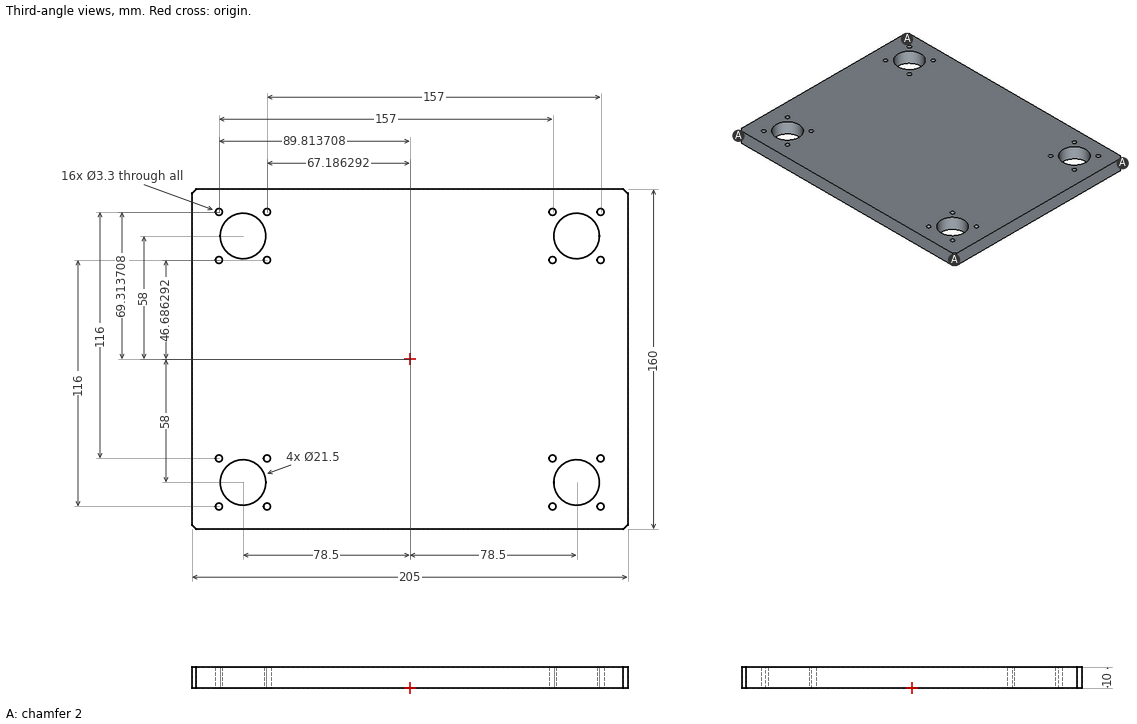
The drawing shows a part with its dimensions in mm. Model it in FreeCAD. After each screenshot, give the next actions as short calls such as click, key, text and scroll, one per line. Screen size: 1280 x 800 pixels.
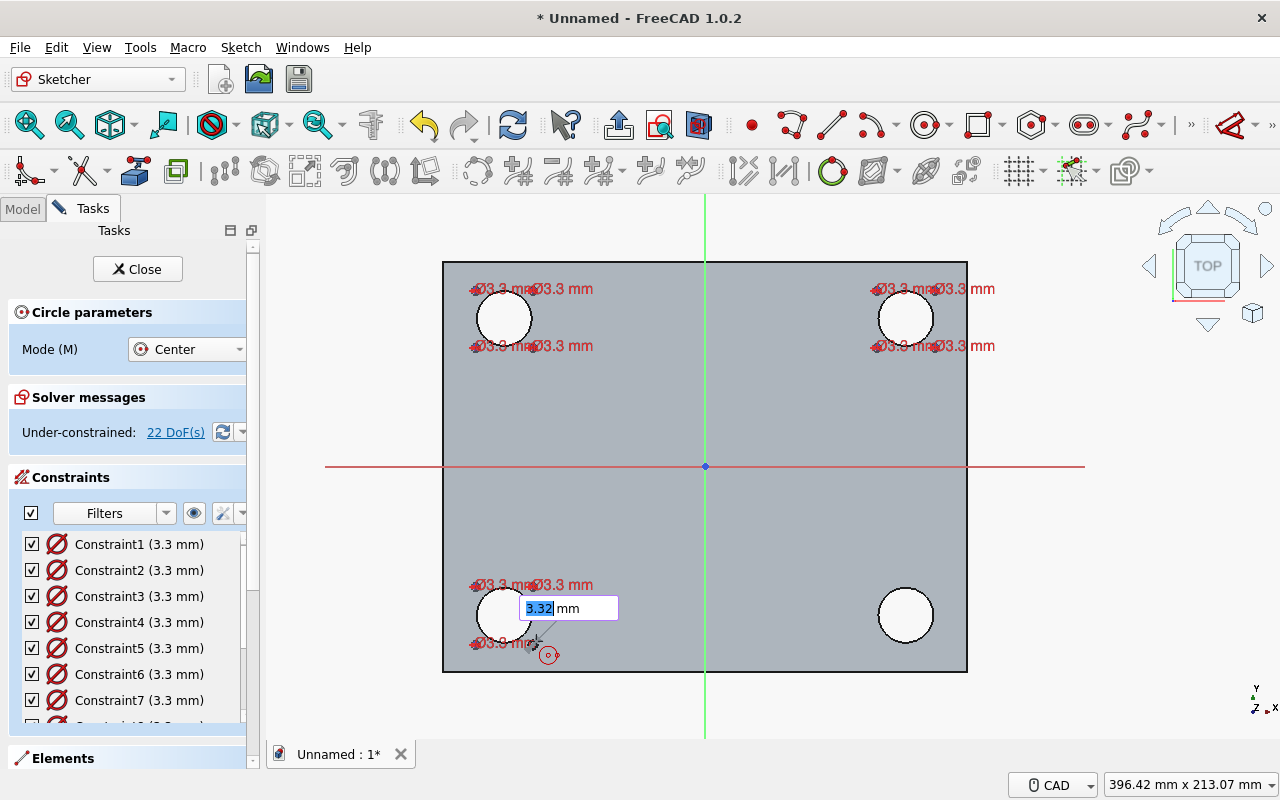
text(3.3)
key(Return)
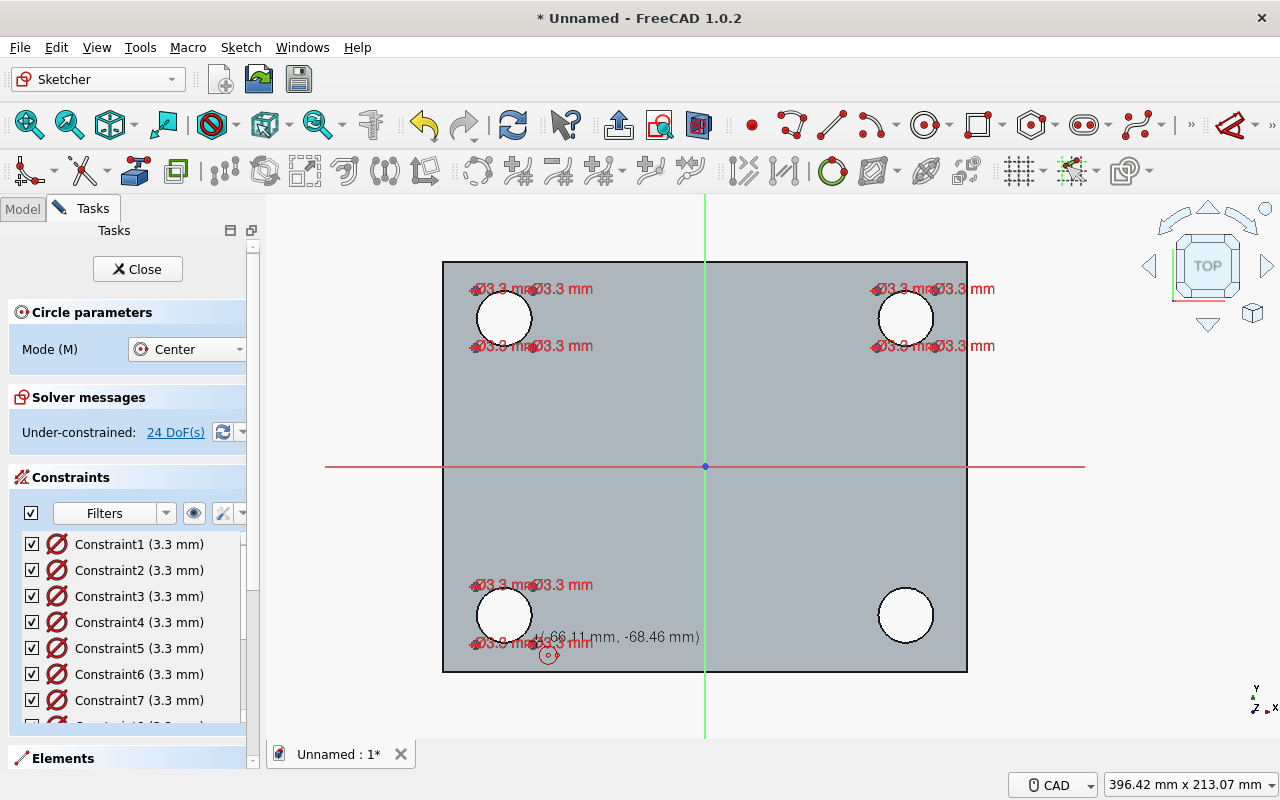
scroll(877, 586, up, 9)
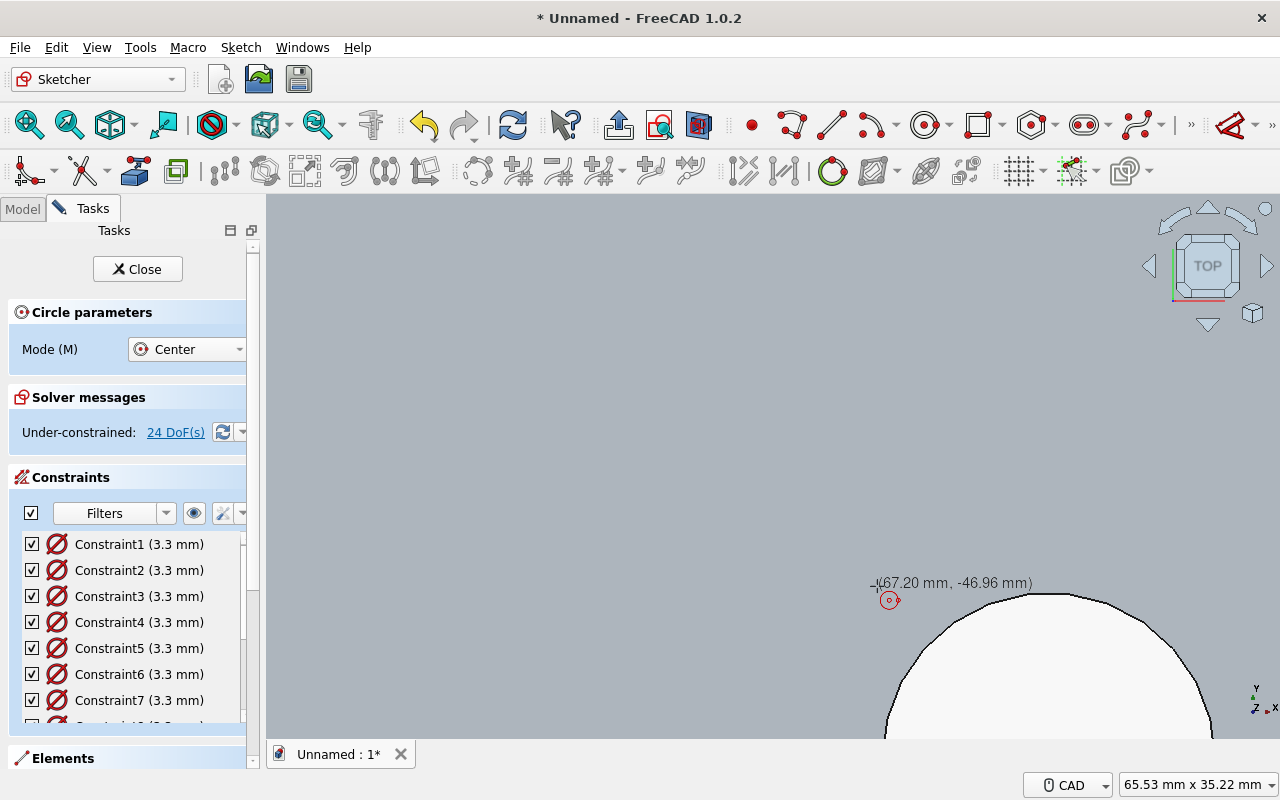
scroll(877, 586, down, 9)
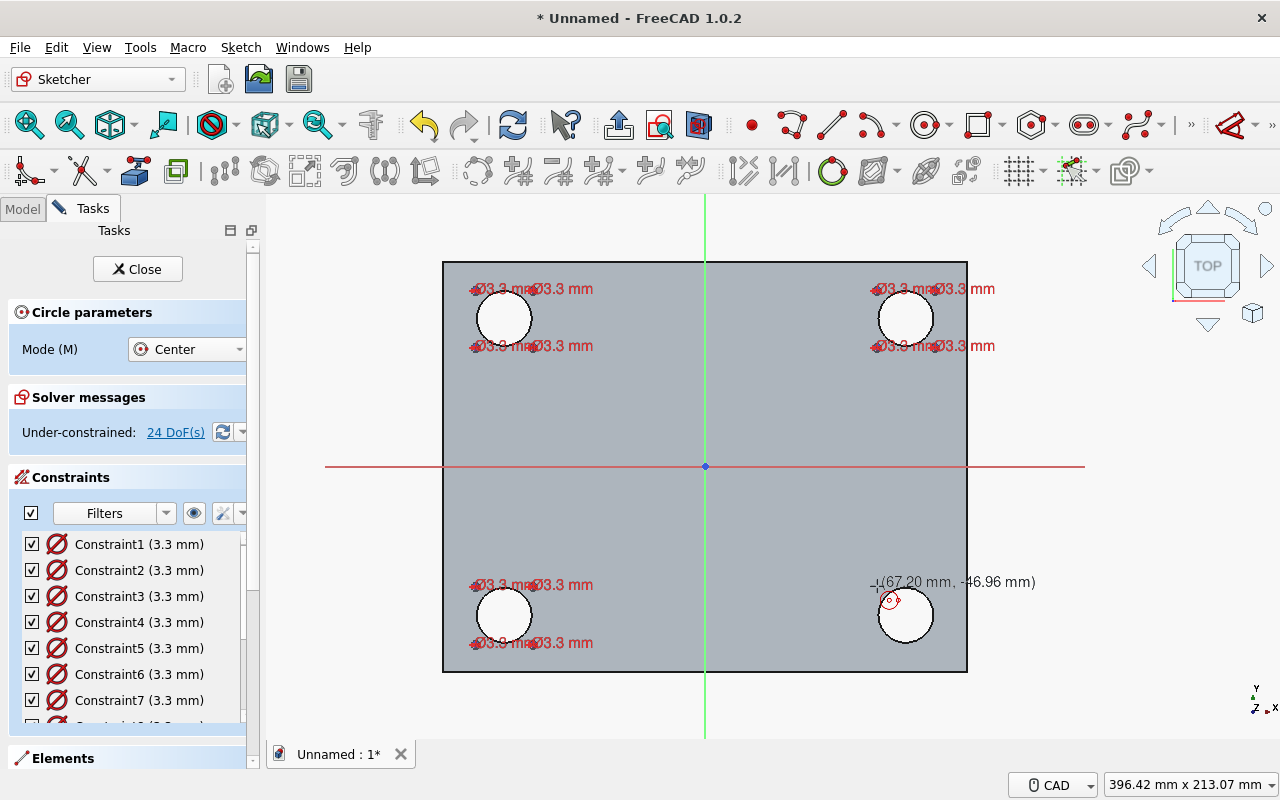
click(877, 586)
move(880, 583)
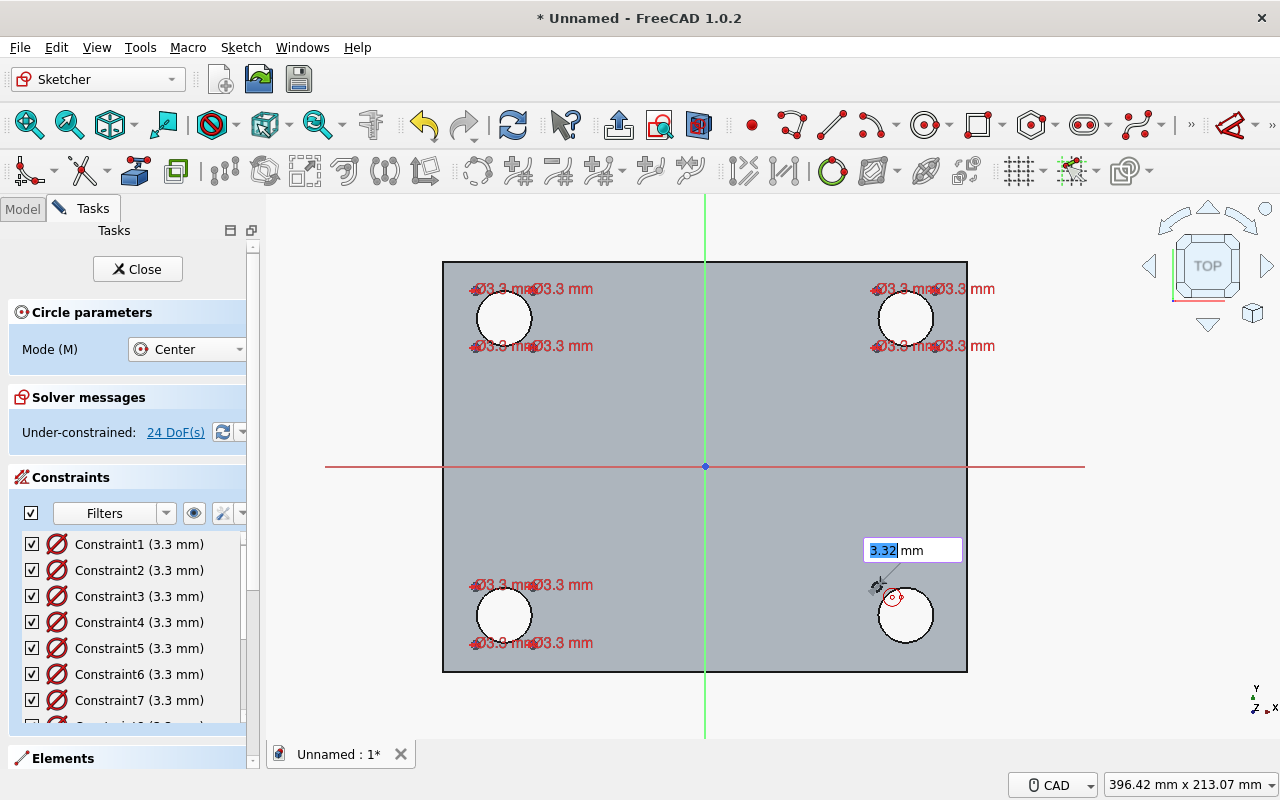
text(3.3)
key(Return)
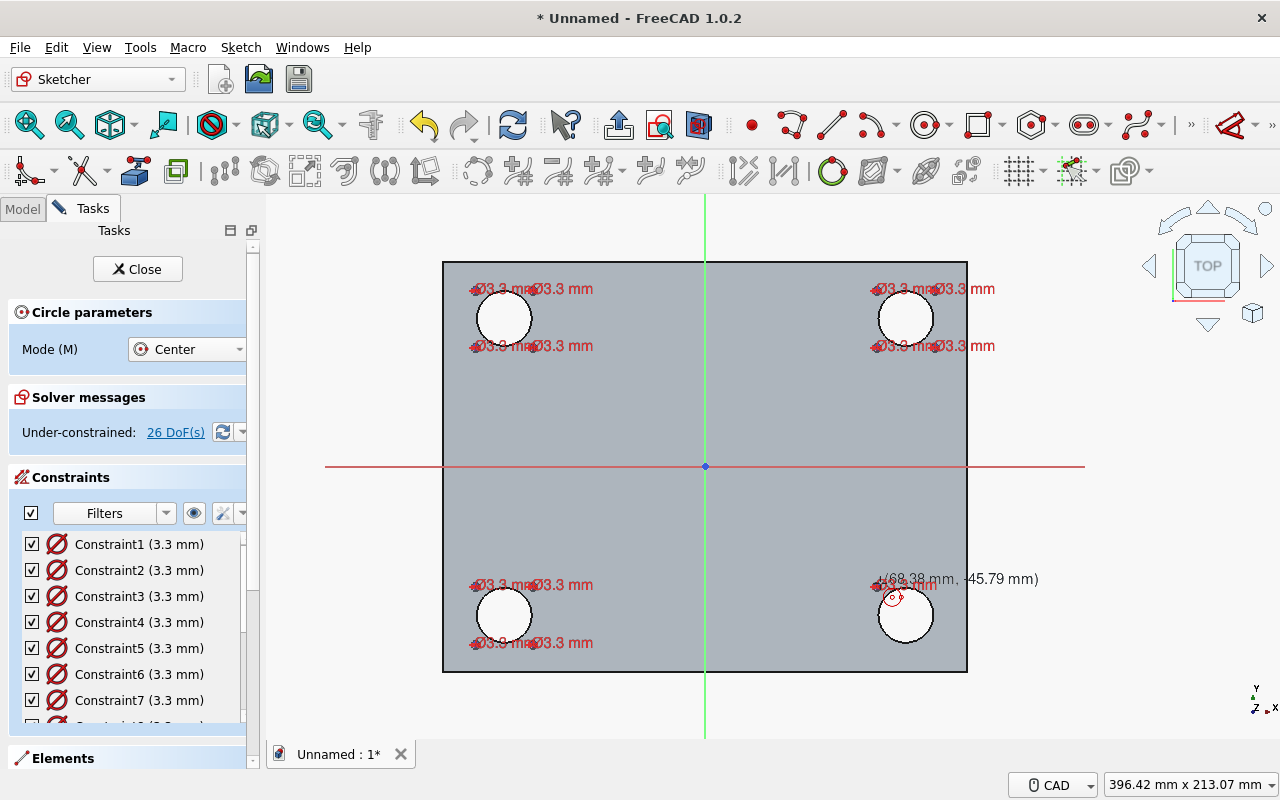
scroll(935, 586, up, 9)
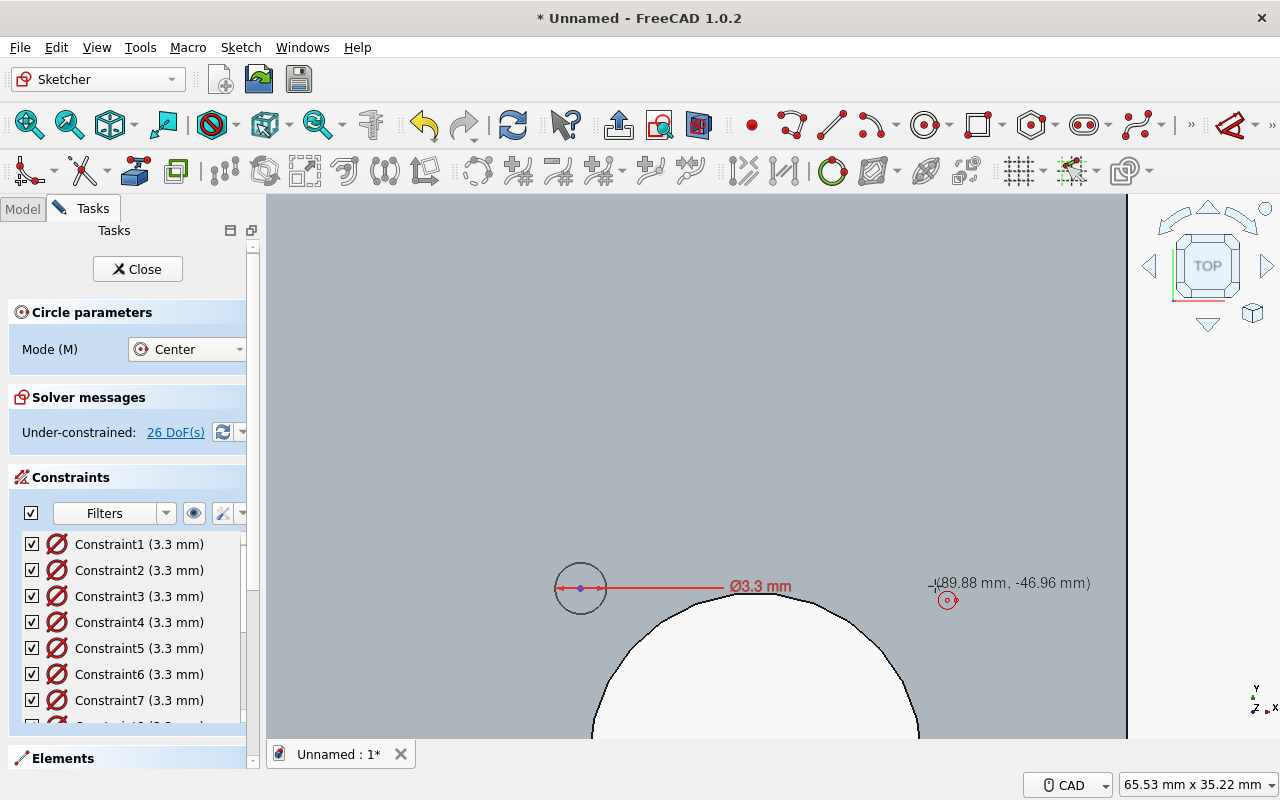
scroll(935, 586, down, 9)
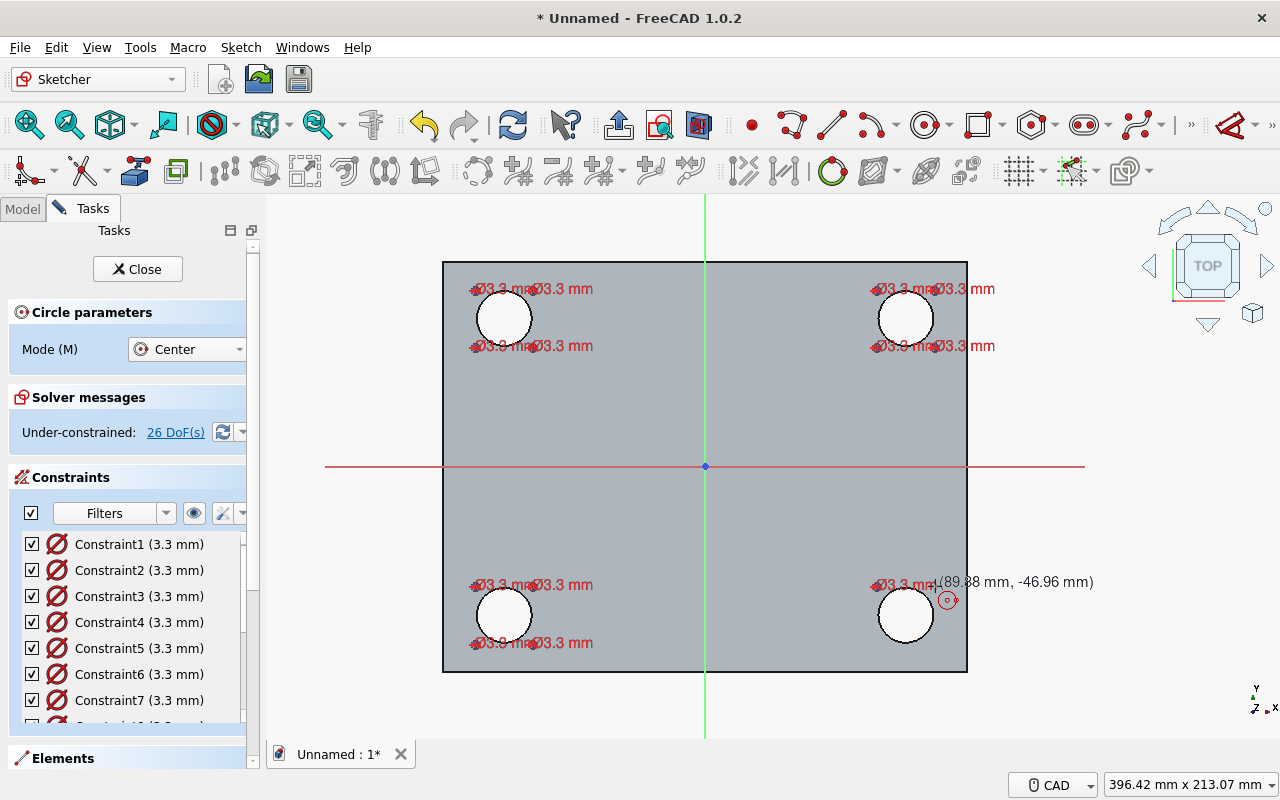
click(935, 586)
move(938, 583)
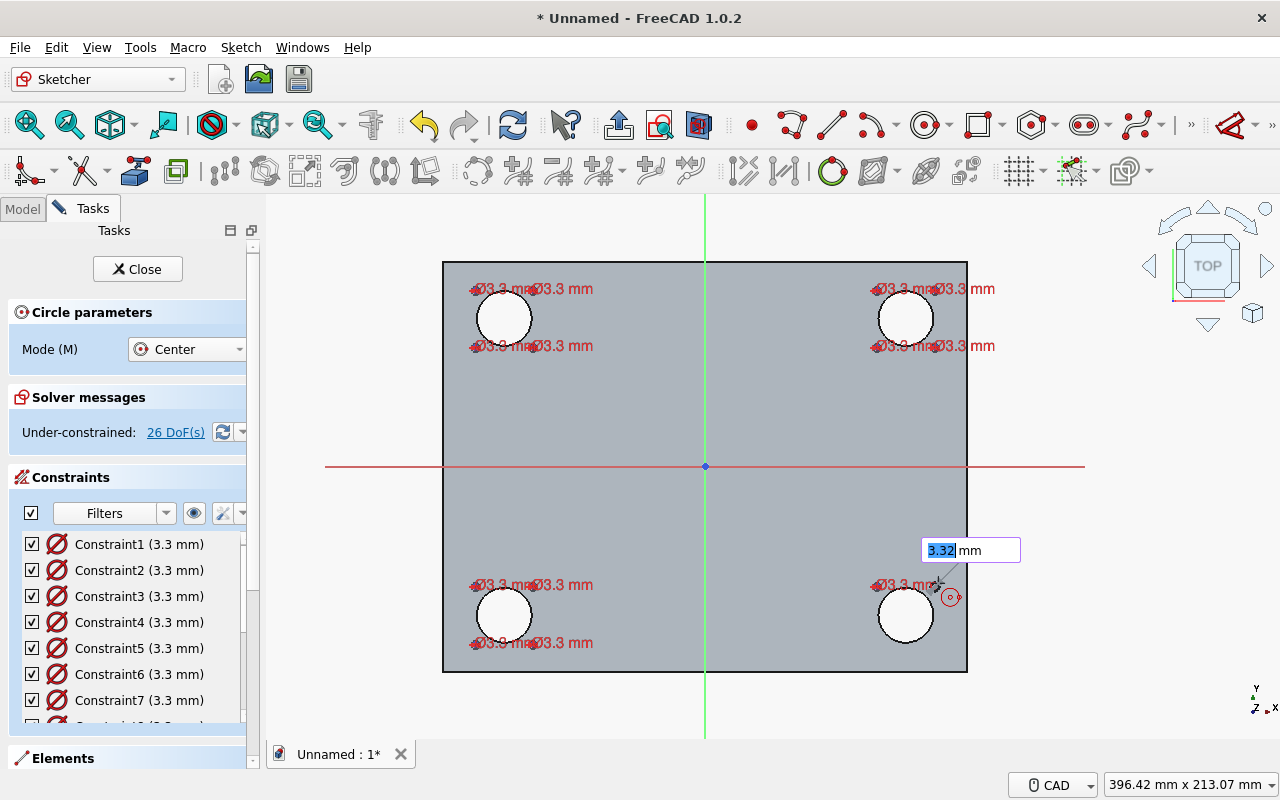
text(3.3)
key(Return)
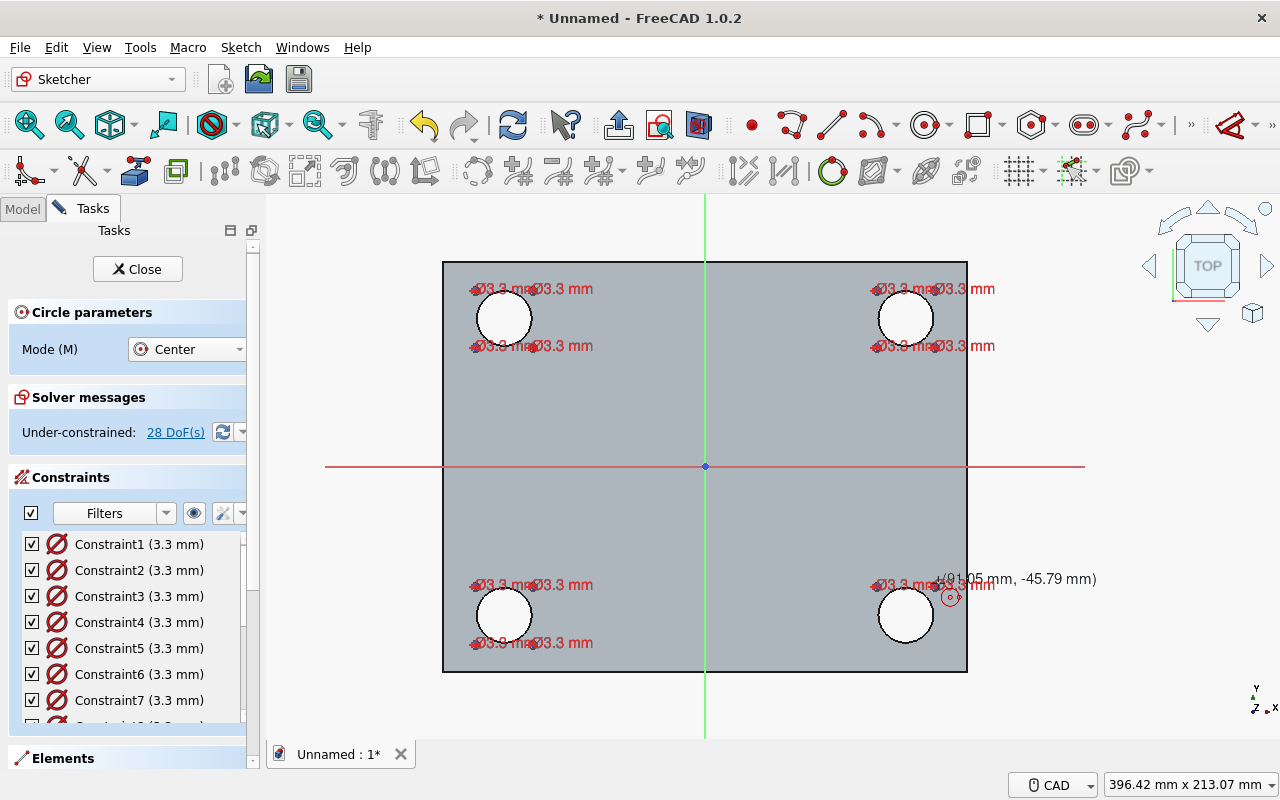
scroll(877, 644, up, 9)